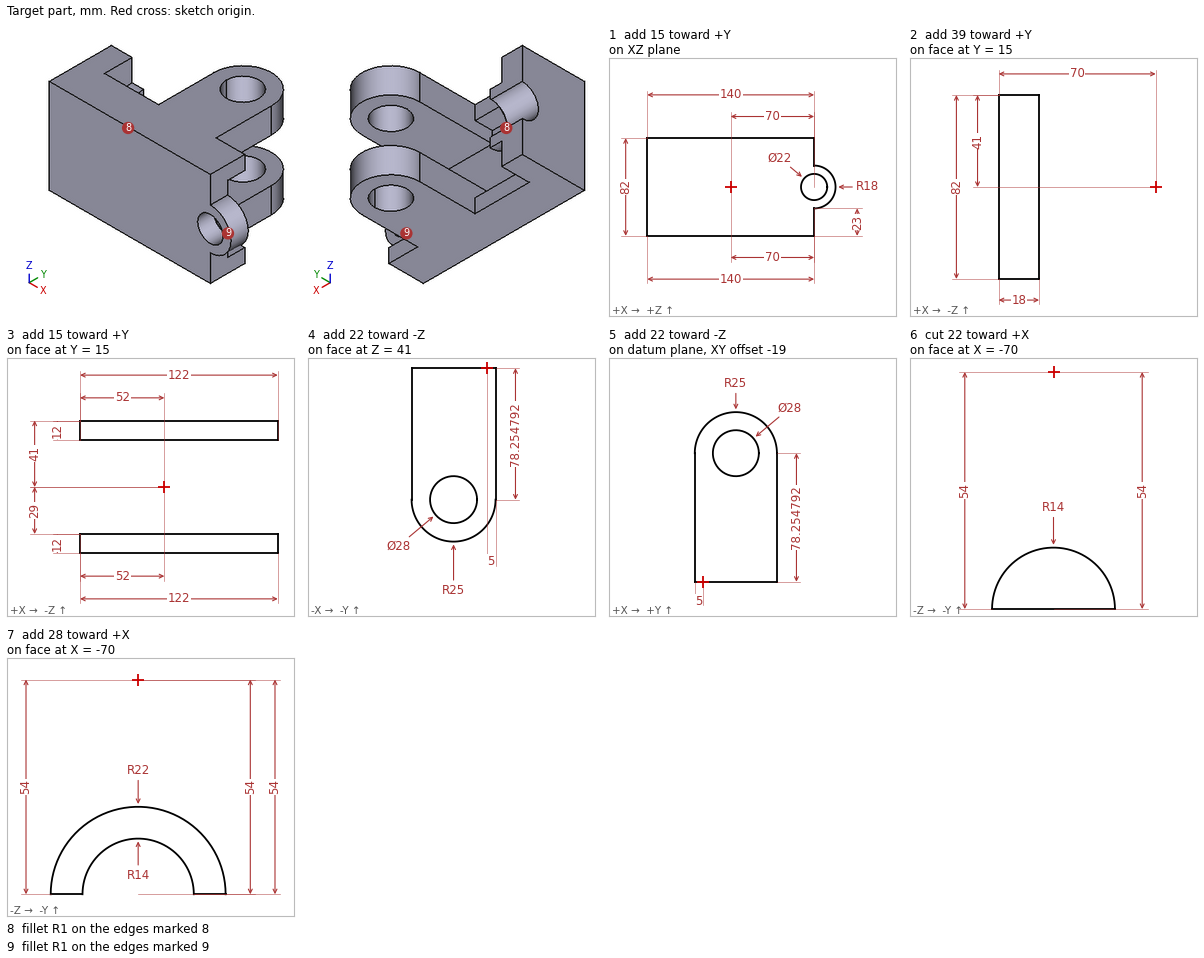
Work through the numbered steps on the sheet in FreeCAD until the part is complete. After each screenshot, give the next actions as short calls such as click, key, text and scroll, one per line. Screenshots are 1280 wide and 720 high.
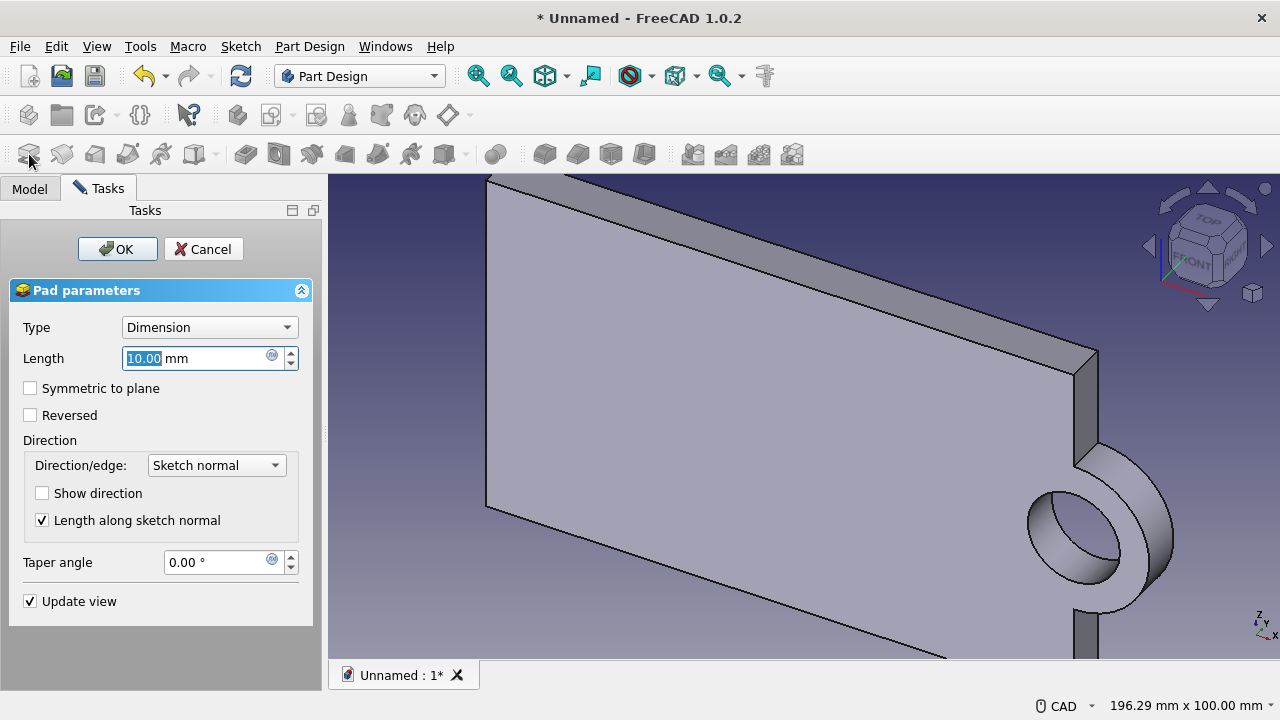
text(15)
key(Tab)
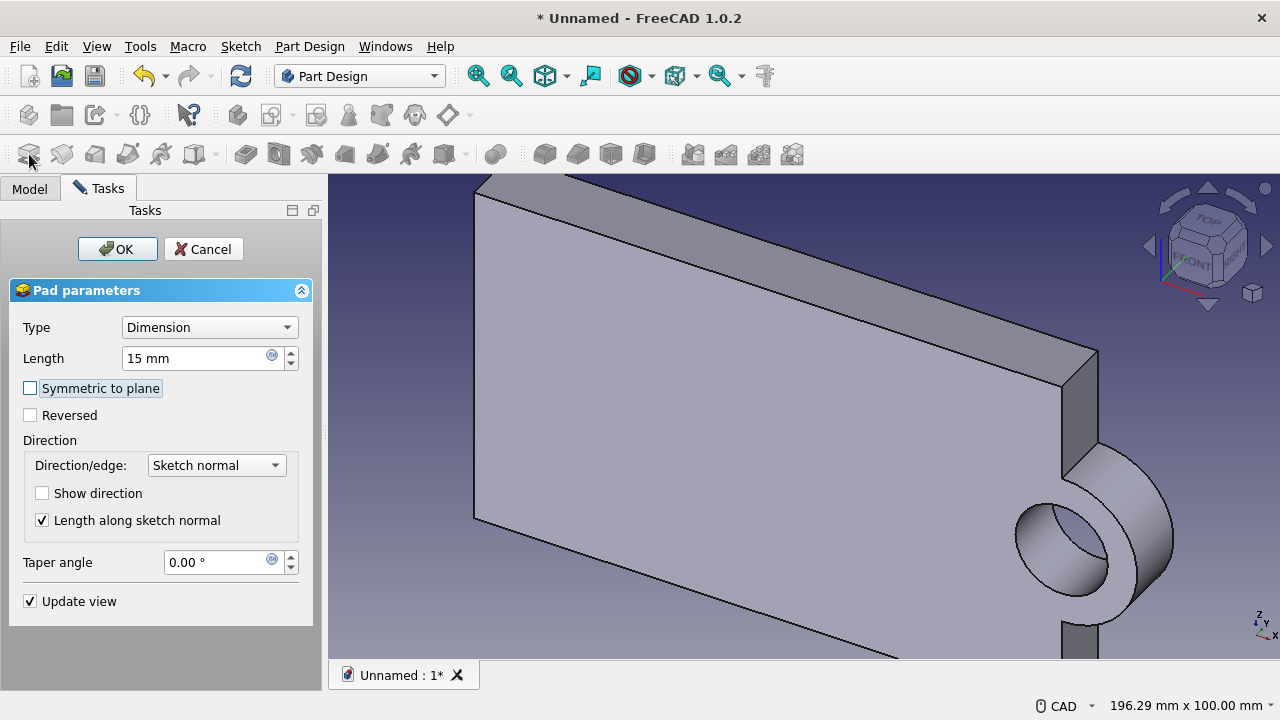
click(31, 415)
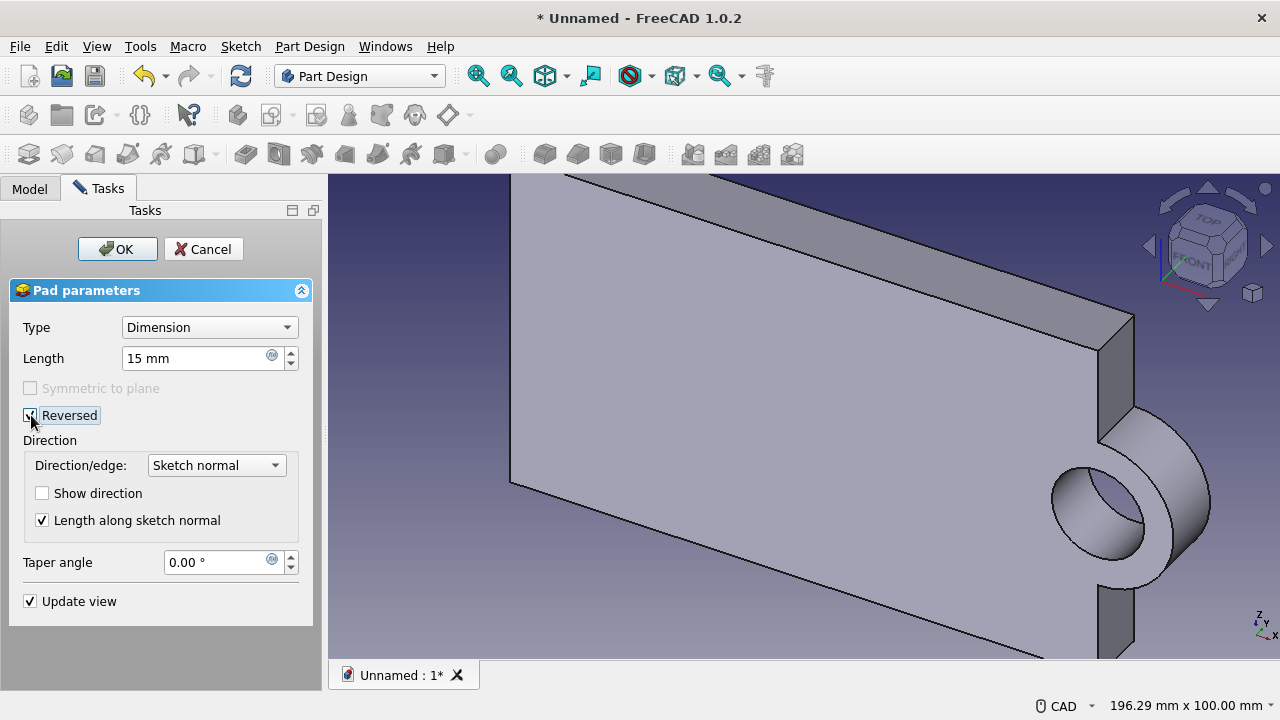
click(118, 249)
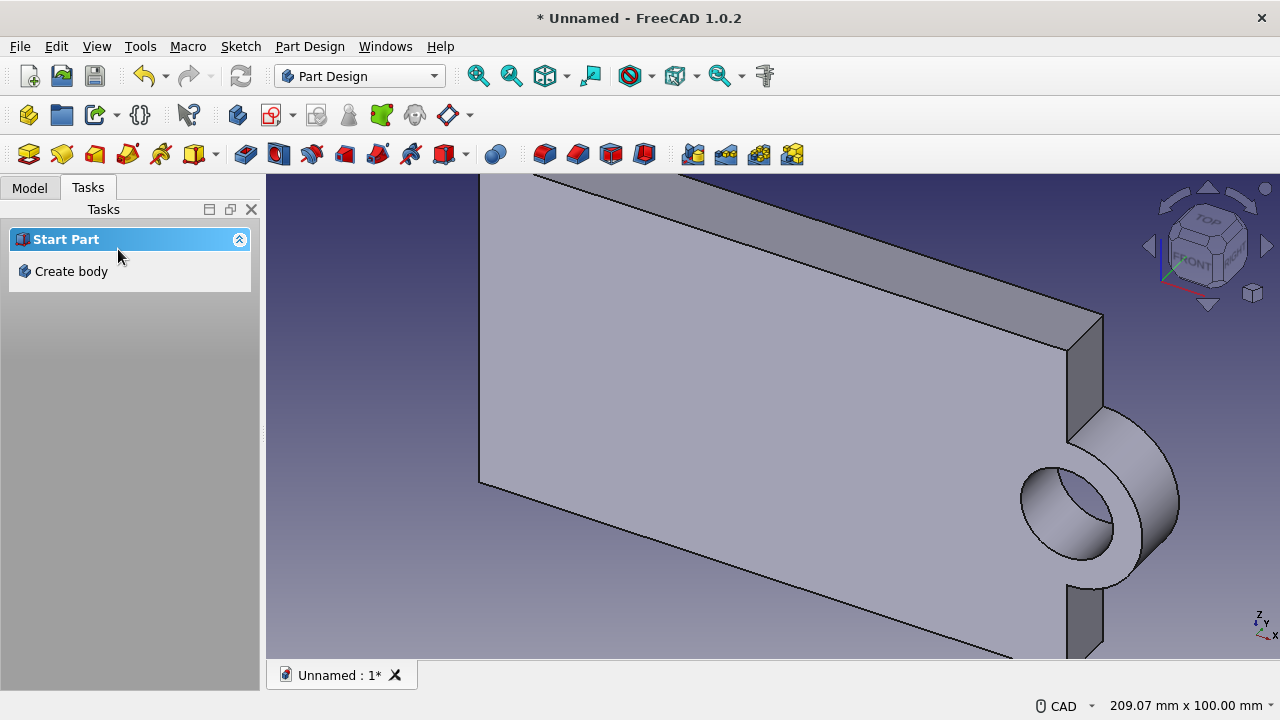
click(479, 76)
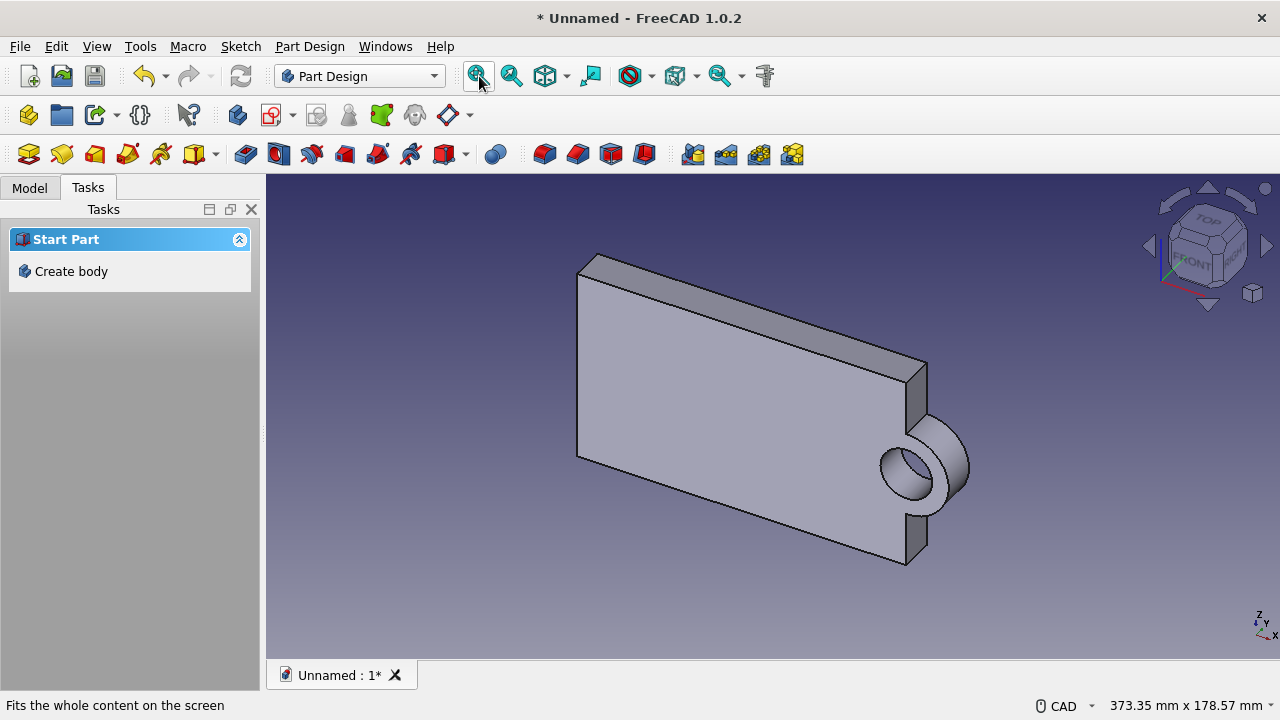
key(4)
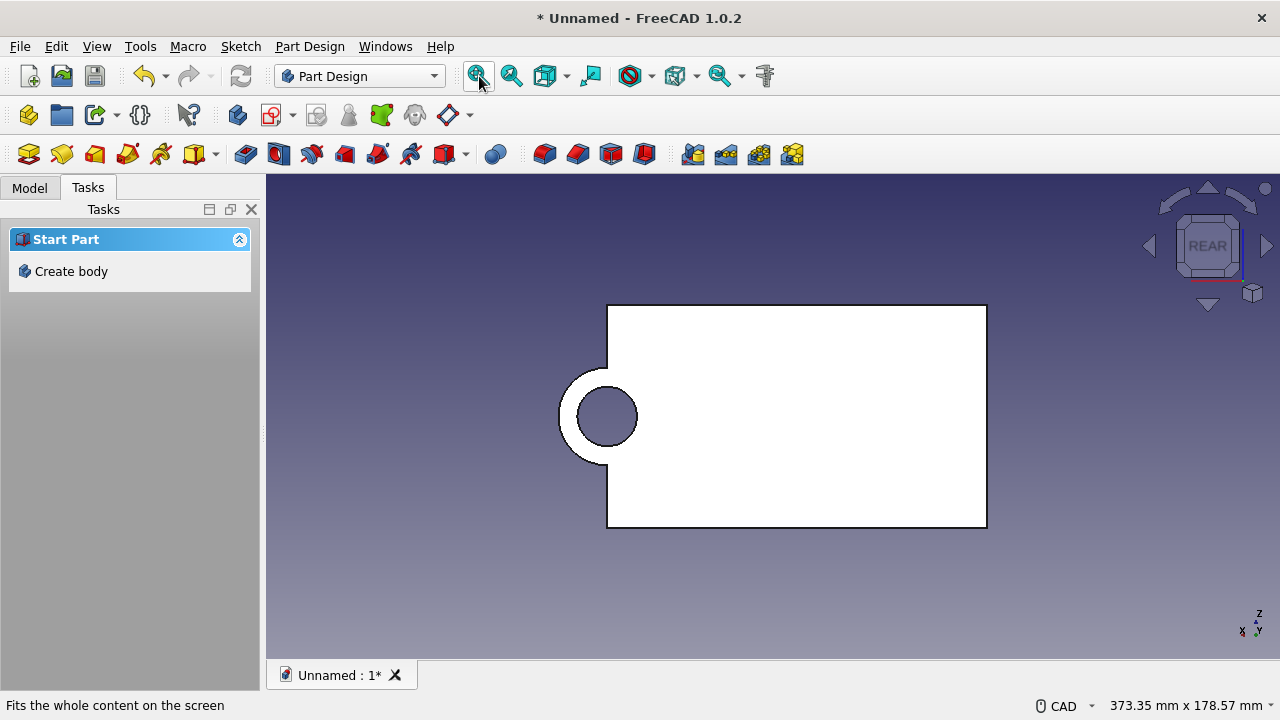
click(773, 416)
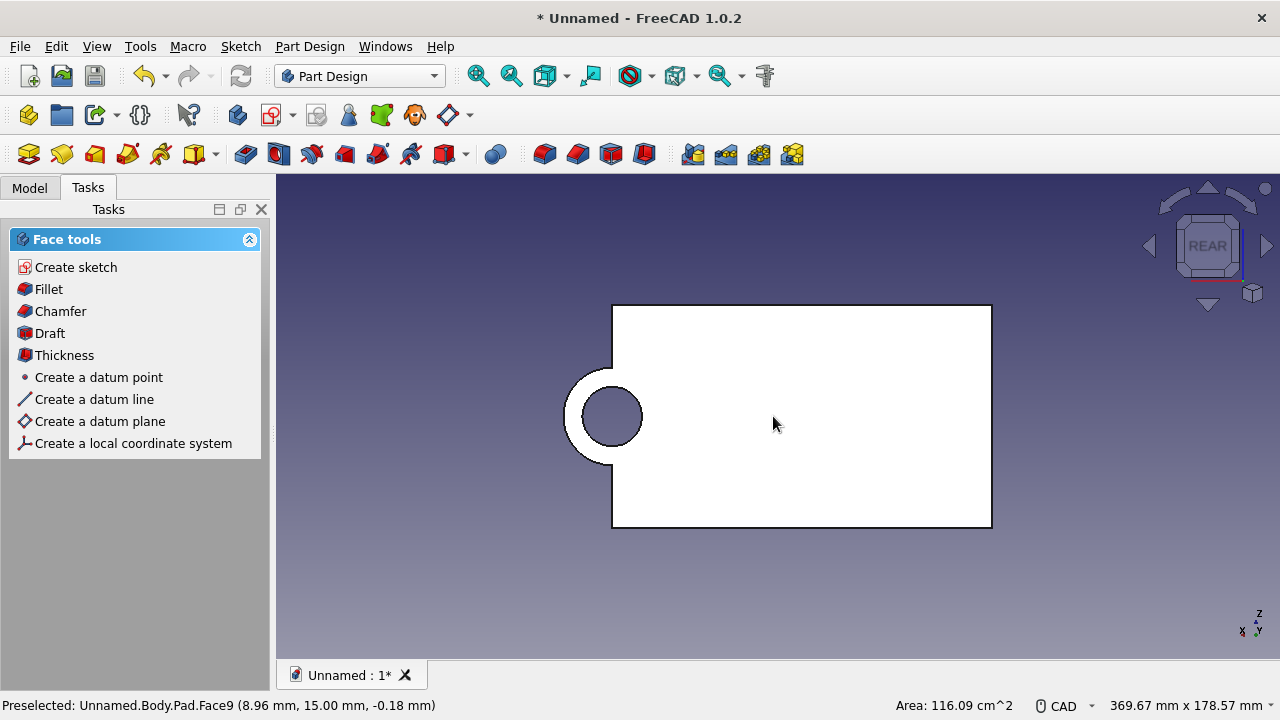
click(270, 116)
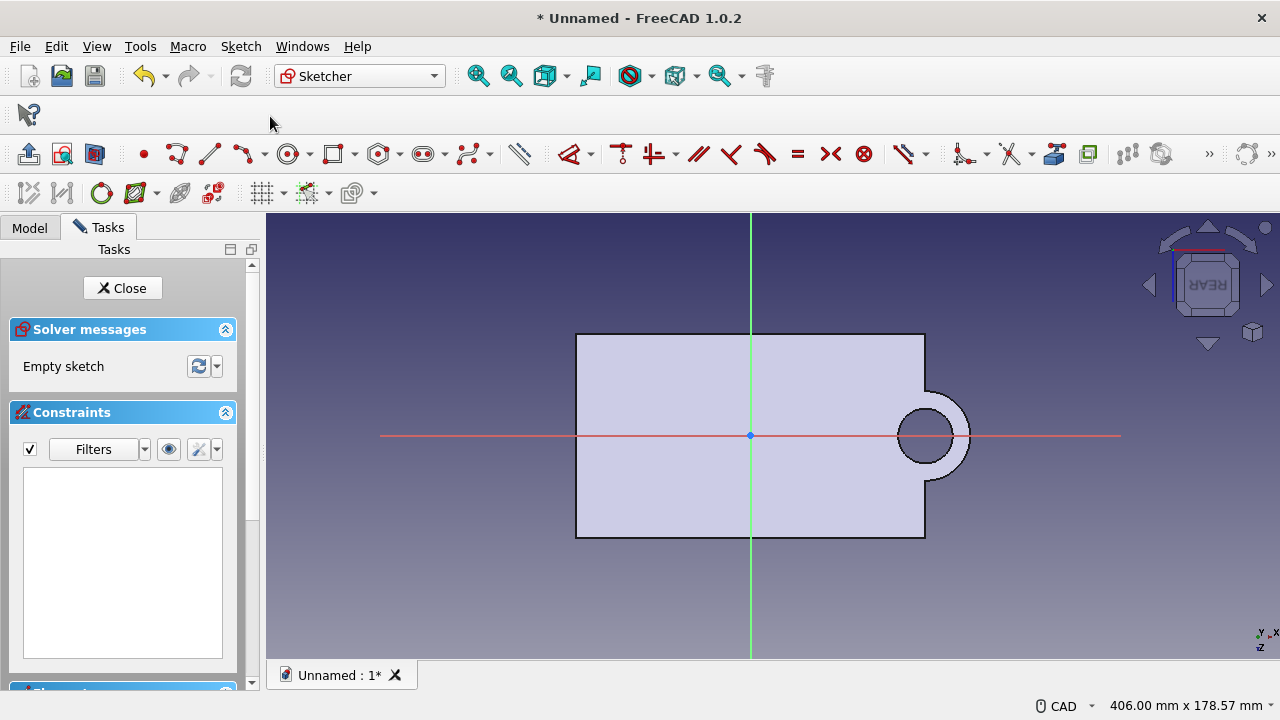
click(332, 154)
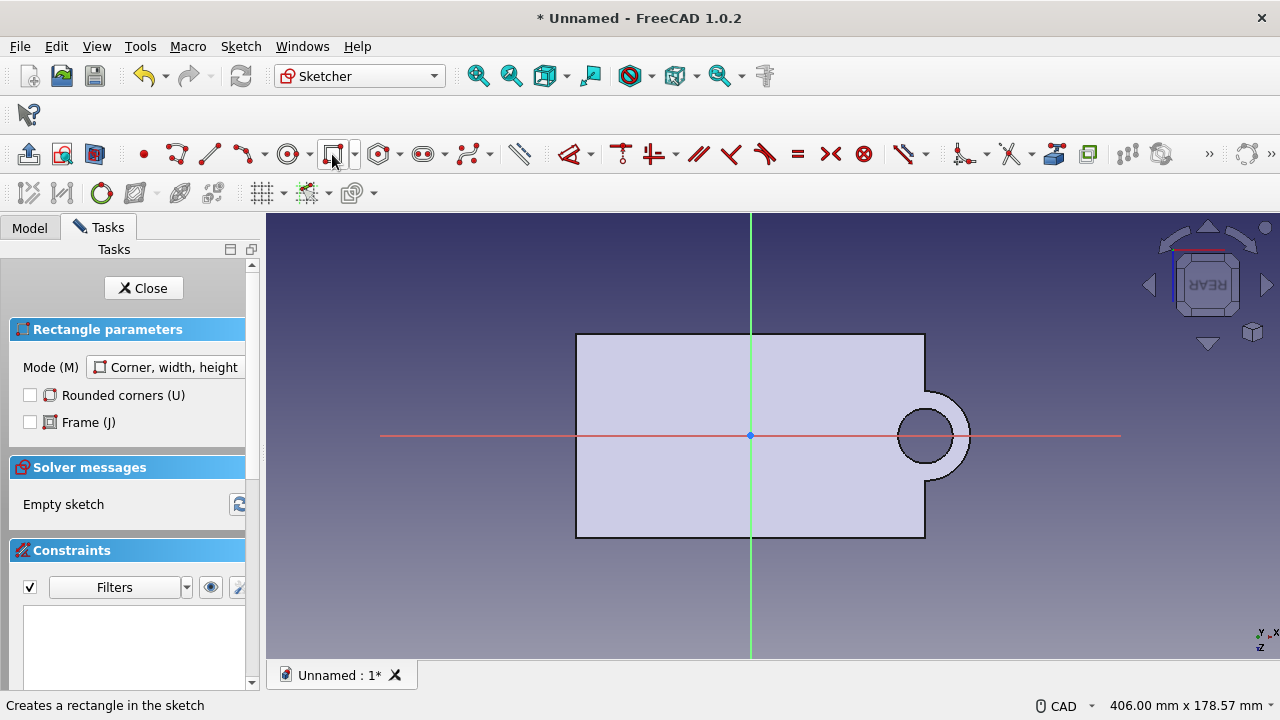
click(576, 334)
click(621, 538)
key(Escape)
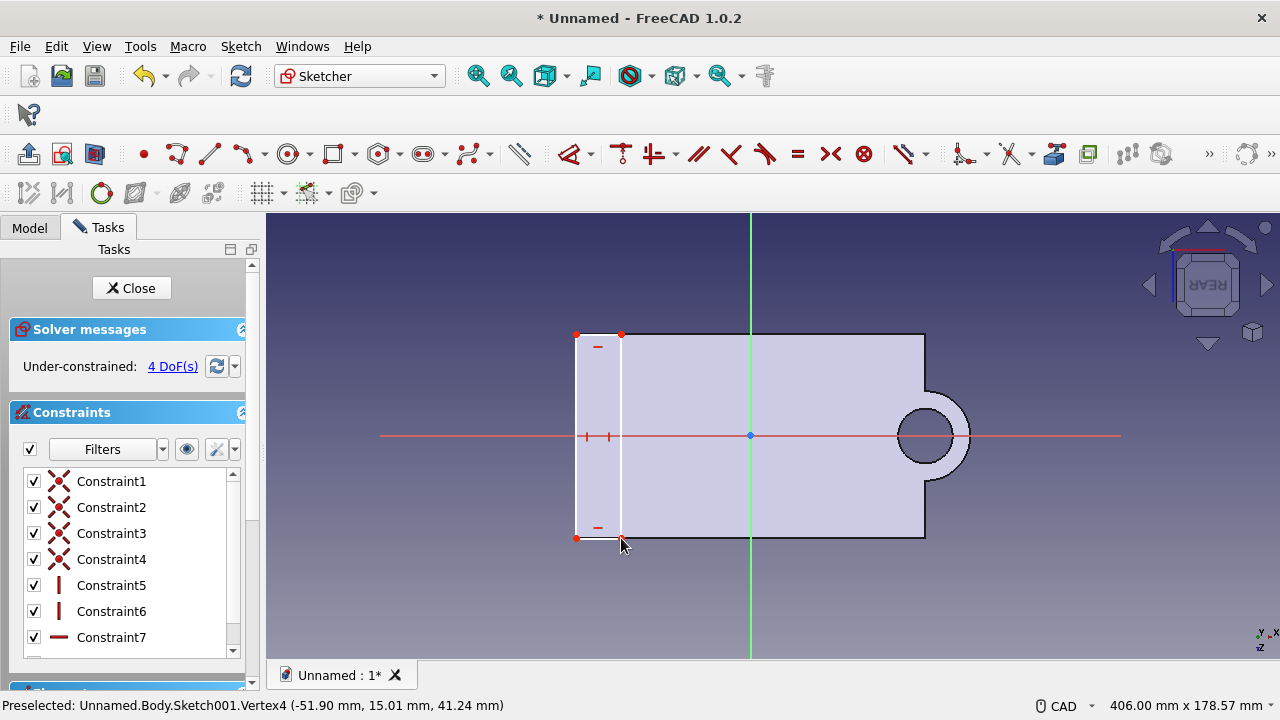
click(568, 154)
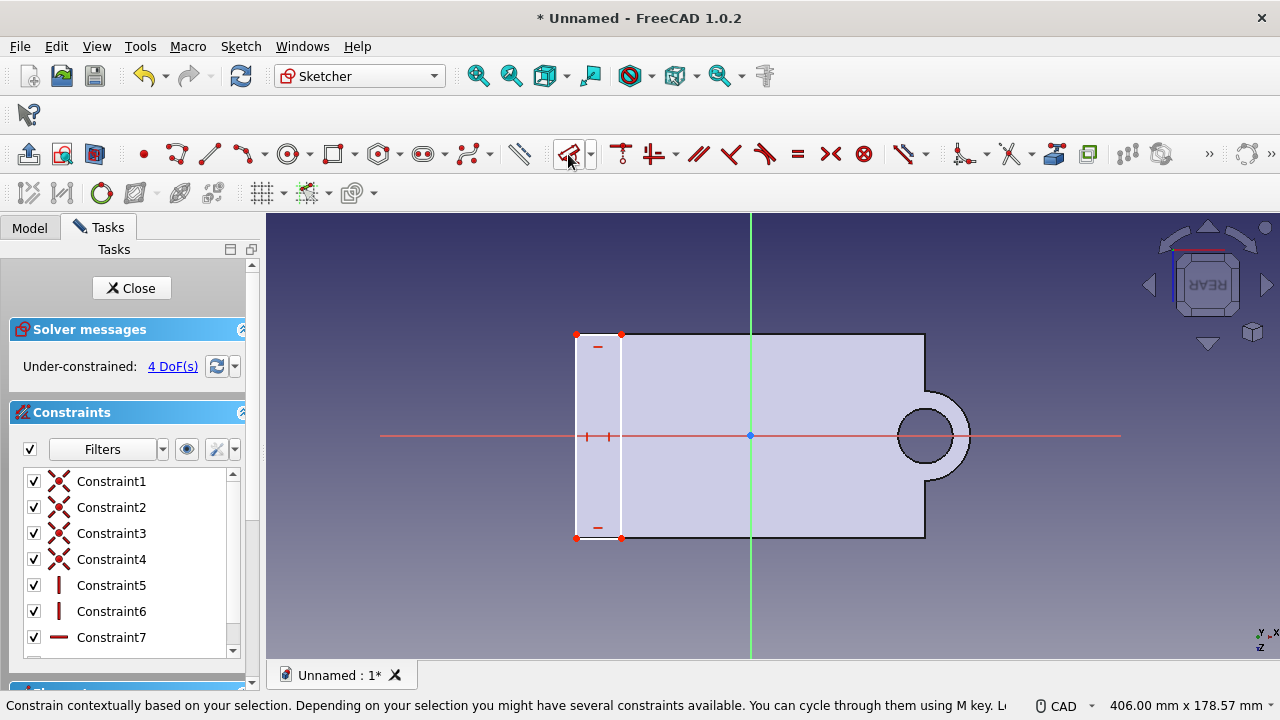
click(576, 396)
click(542, 390)